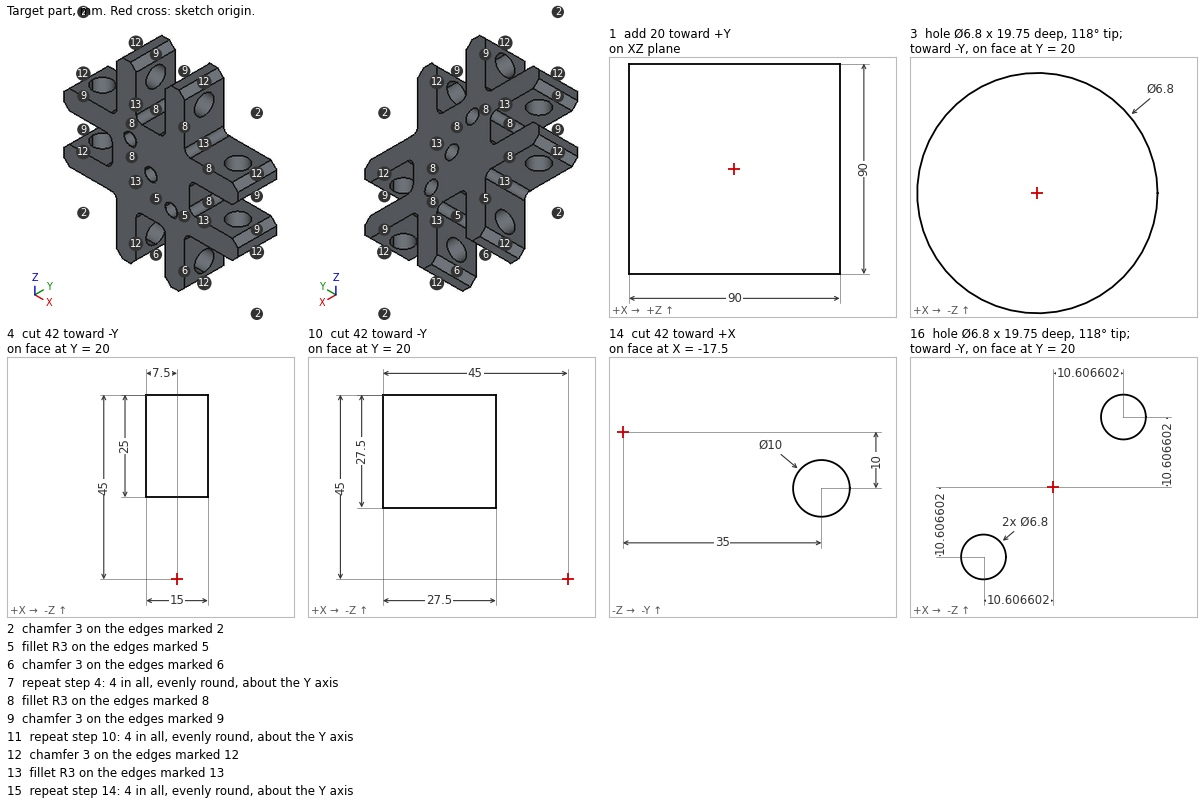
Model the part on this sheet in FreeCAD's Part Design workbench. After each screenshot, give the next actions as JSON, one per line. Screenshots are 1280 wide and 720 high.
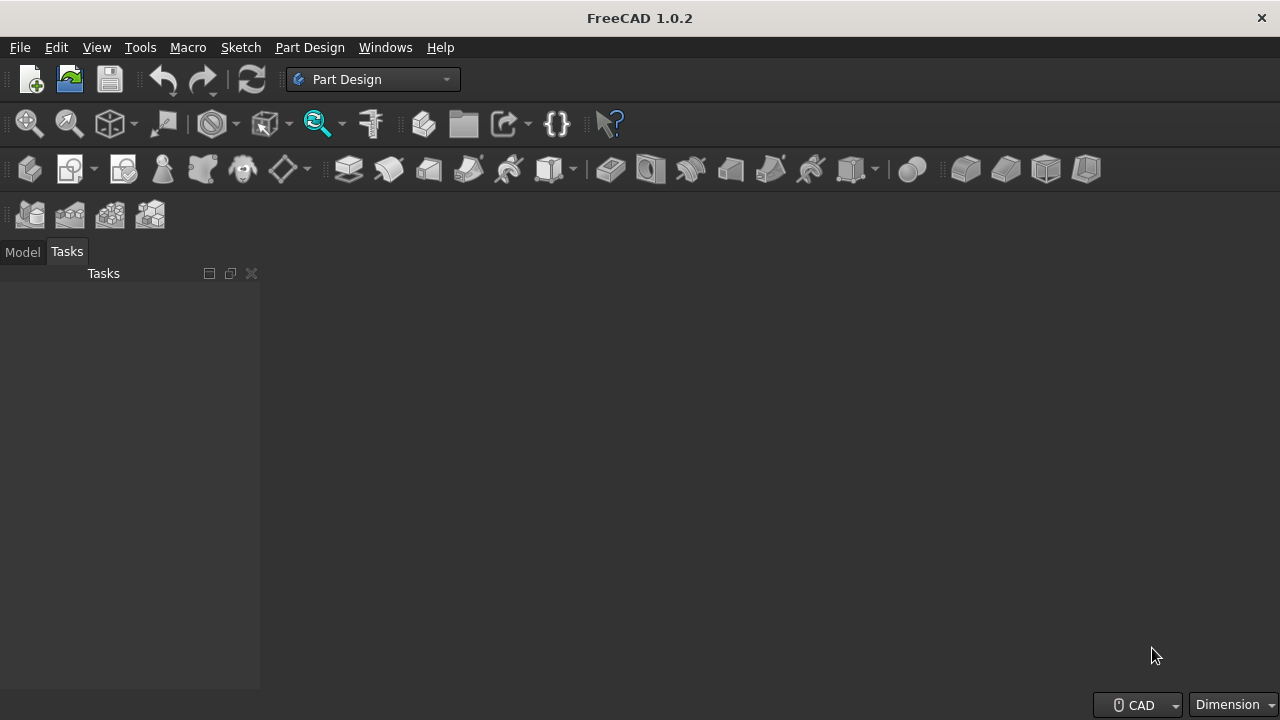
{"action": "left_click", "coordinate": [30, 80]}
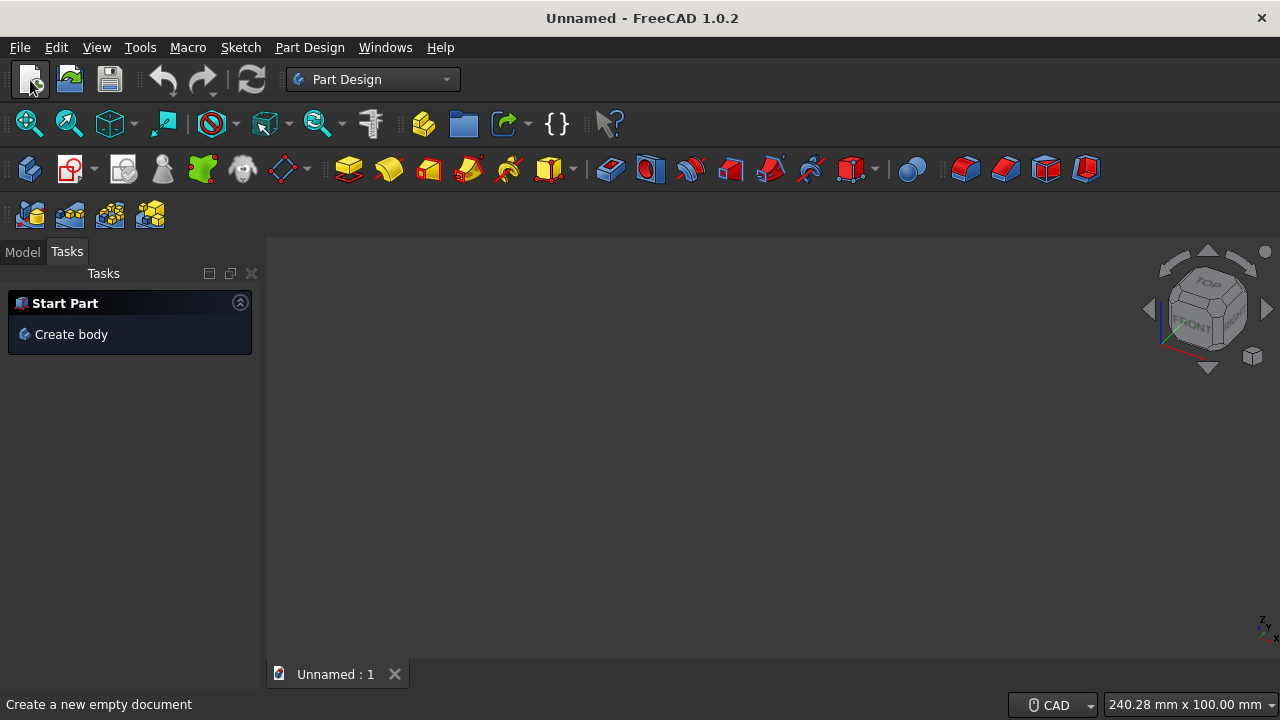
{"action": "left_click", "coordinate": [70, 170]}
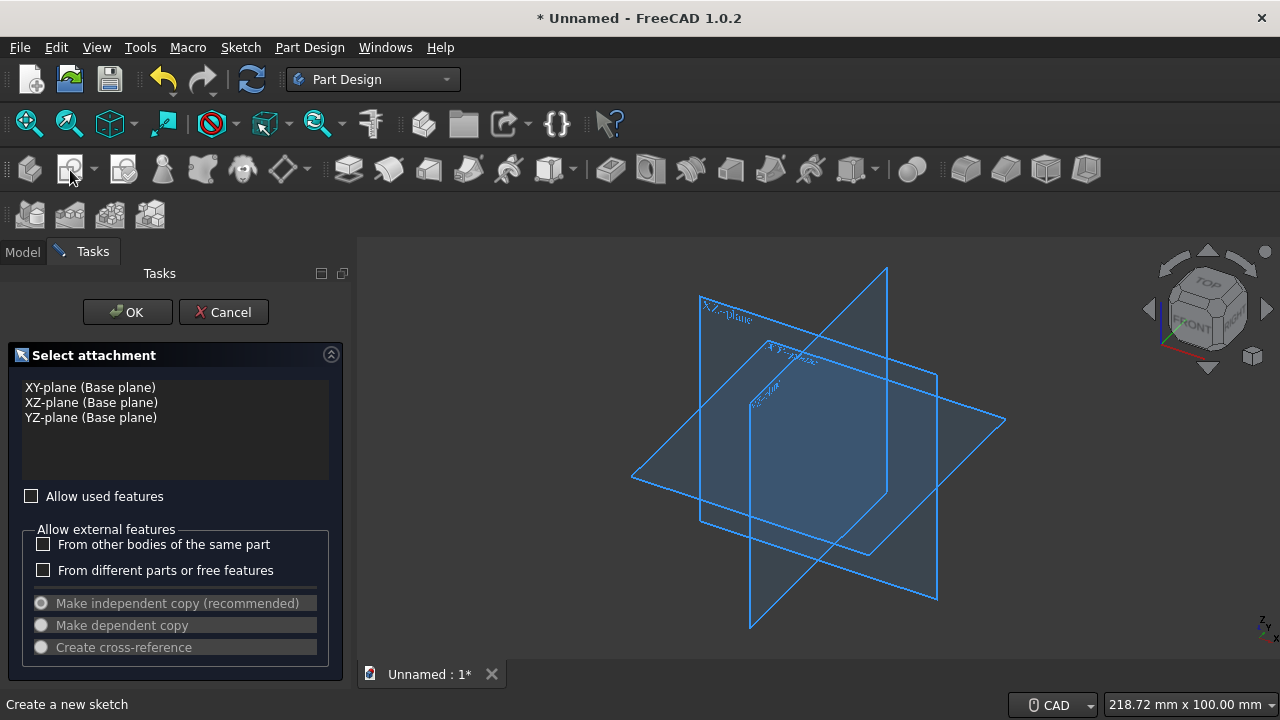
{"action": "left_click", "coordinate": [82, 402]}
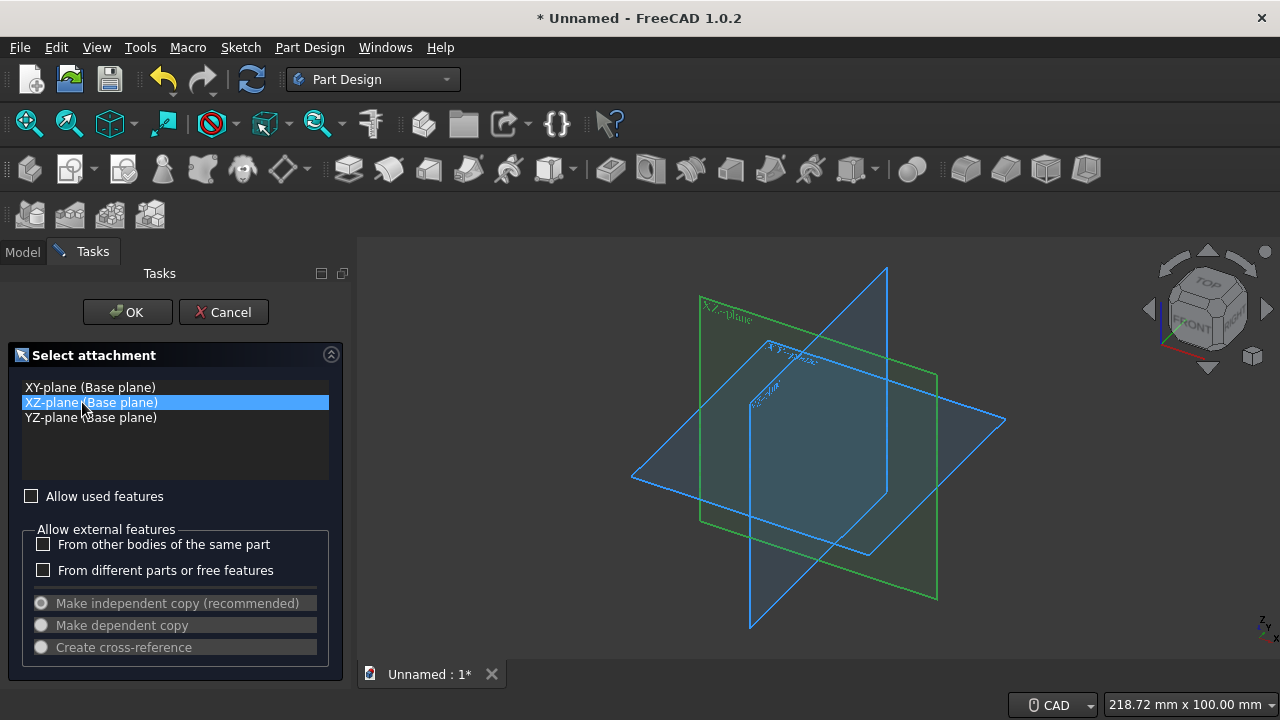
{"action": "left_click", "coordinate": [128, 312]}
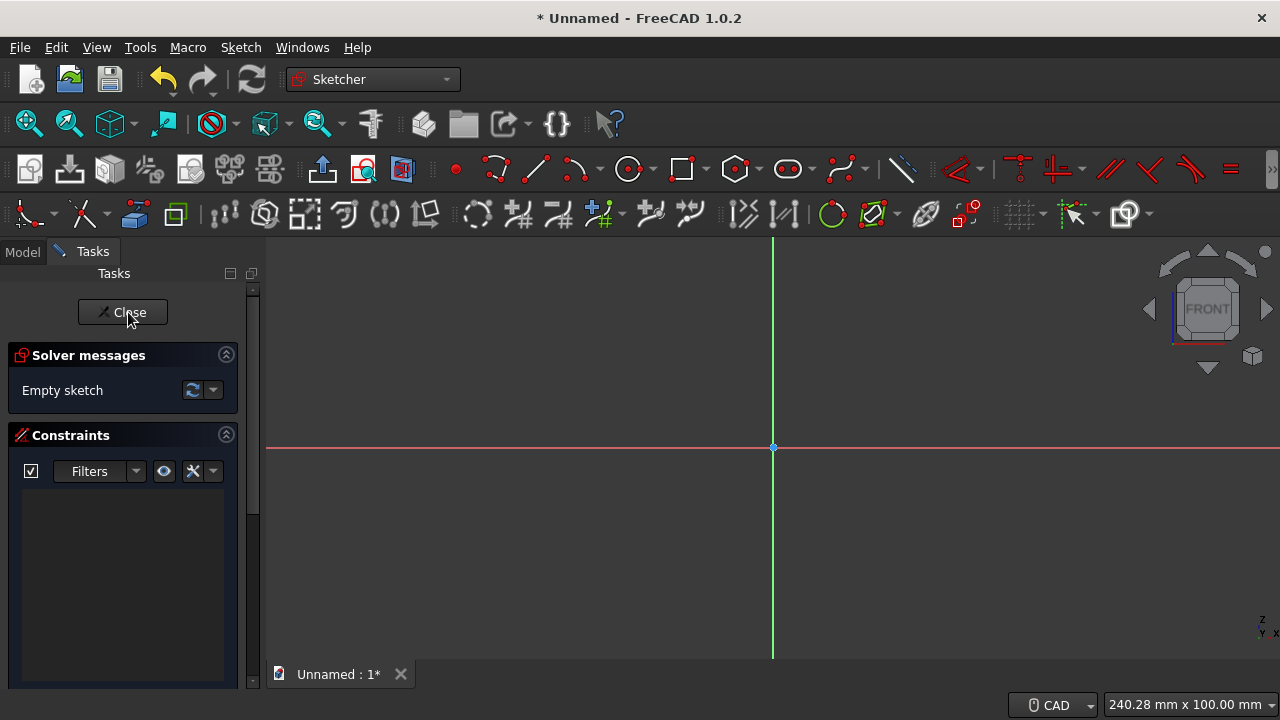
{"action": "scroll", "coordinate": [565, 448], "scroll_direction": "down", "scroll_amount": 2}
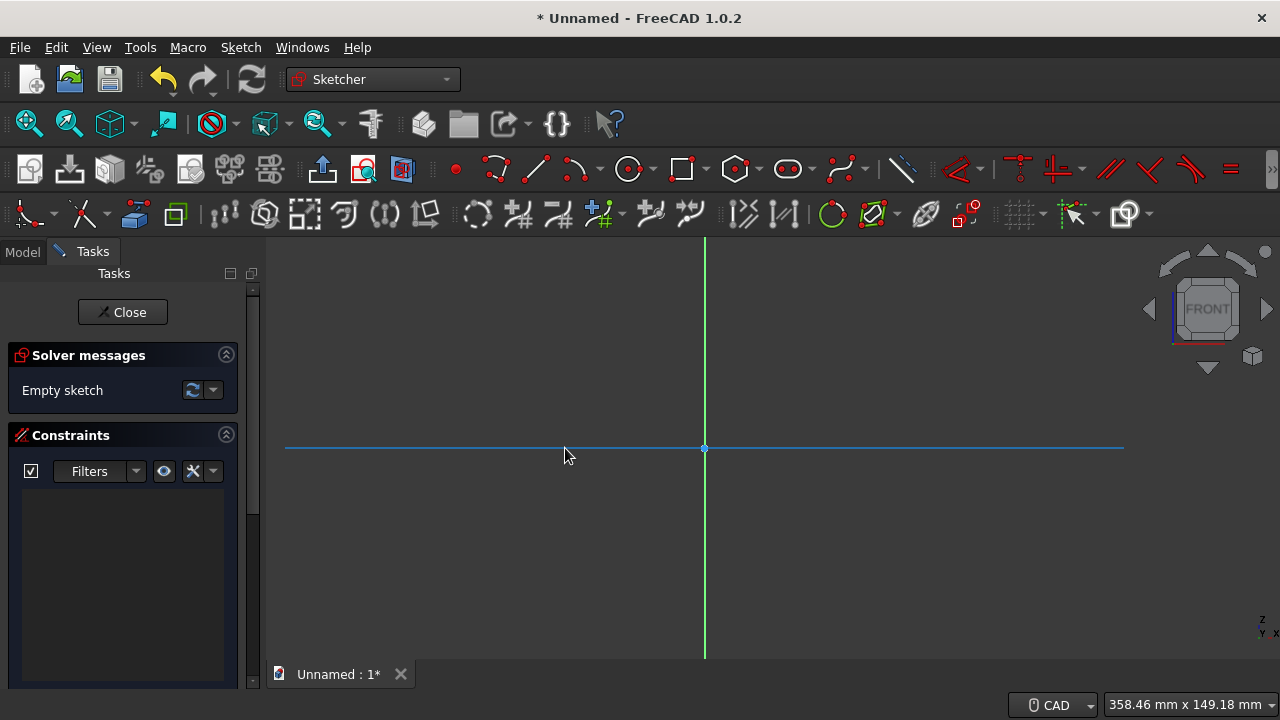
{"action": "left_click", "coordinate": [708, 170]}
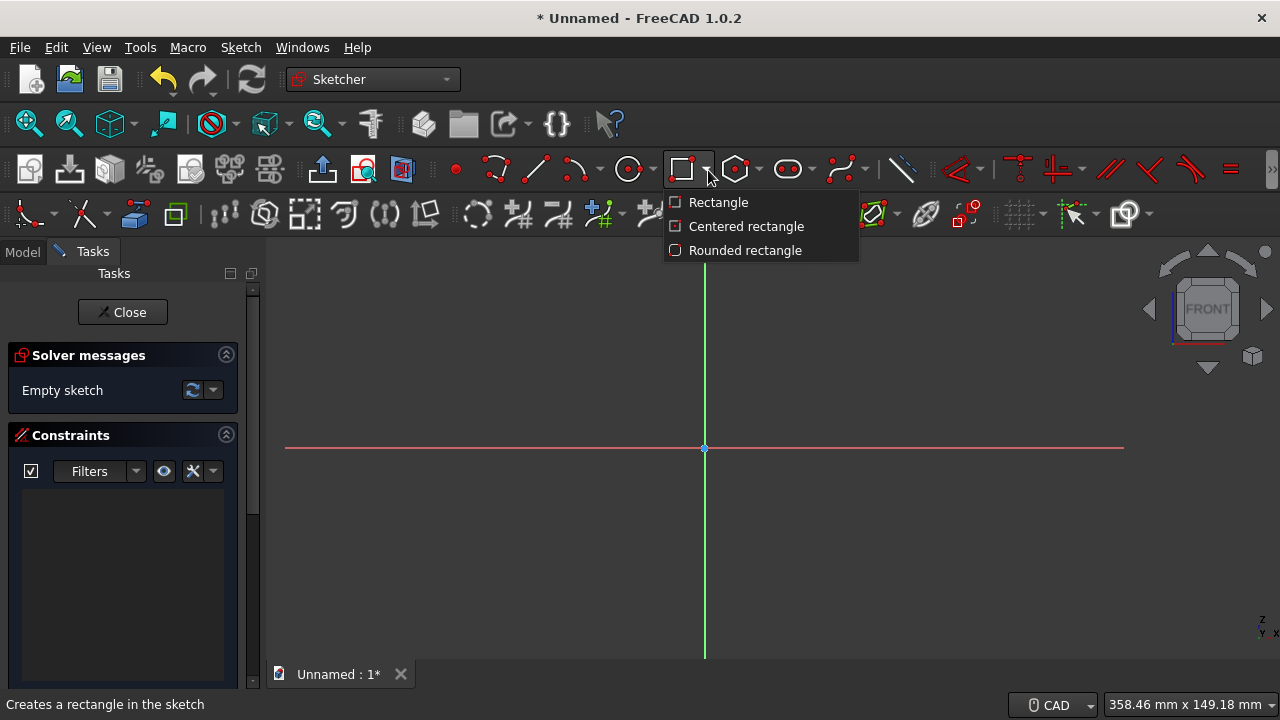
{"action": "left_click", "coordinate": [762, 226]}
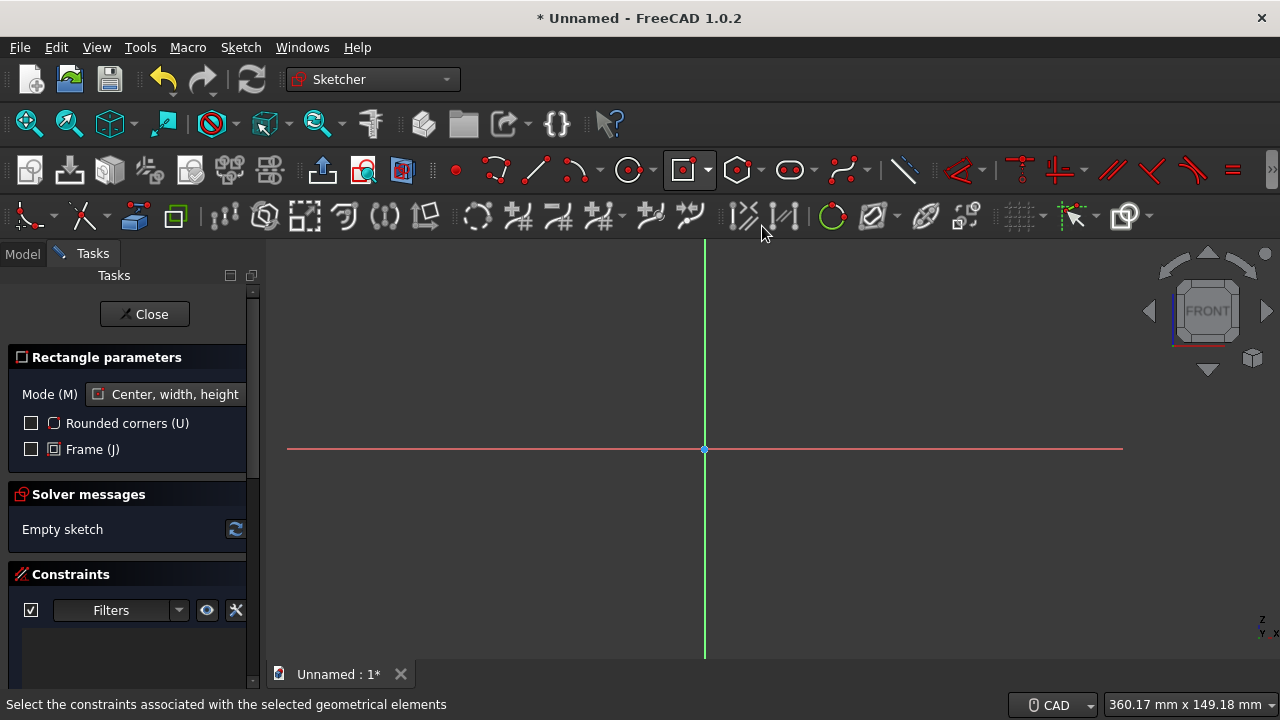
{"action": "left_click", "coordinate": [705, 449]}
{"action": "left_click", "coordinate": [832, 322]}
{"action": "key", "text": "Escape"}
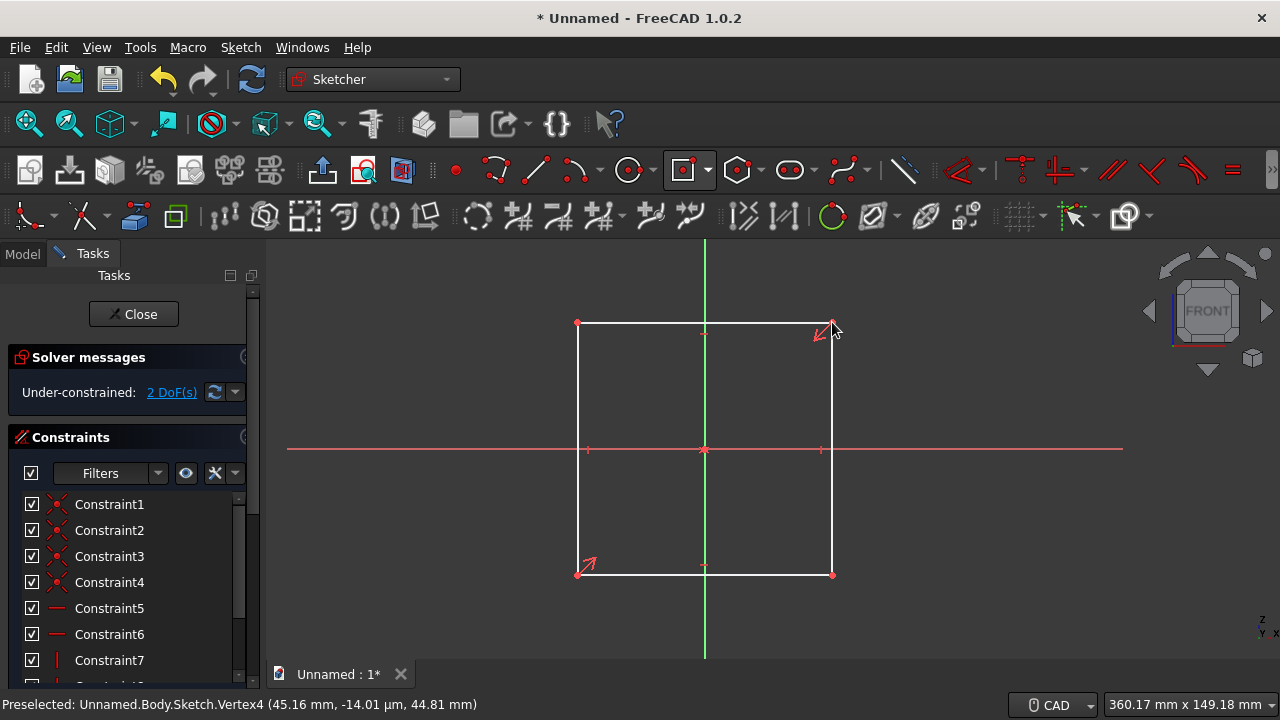
{"action": "left_click", "coordinate": [958, 170]}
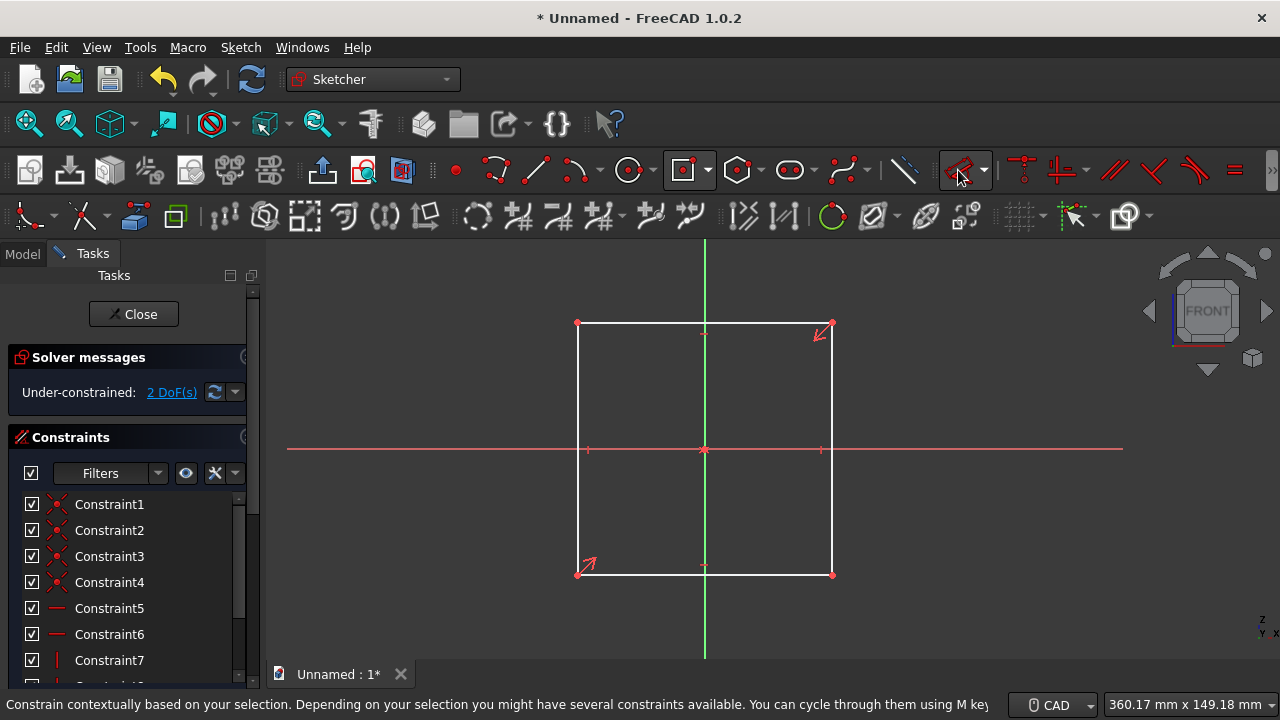
{"action": "left_click", "coordinate": [654, 575]}
{"action": "left_click", "coordinate": [646, 609]}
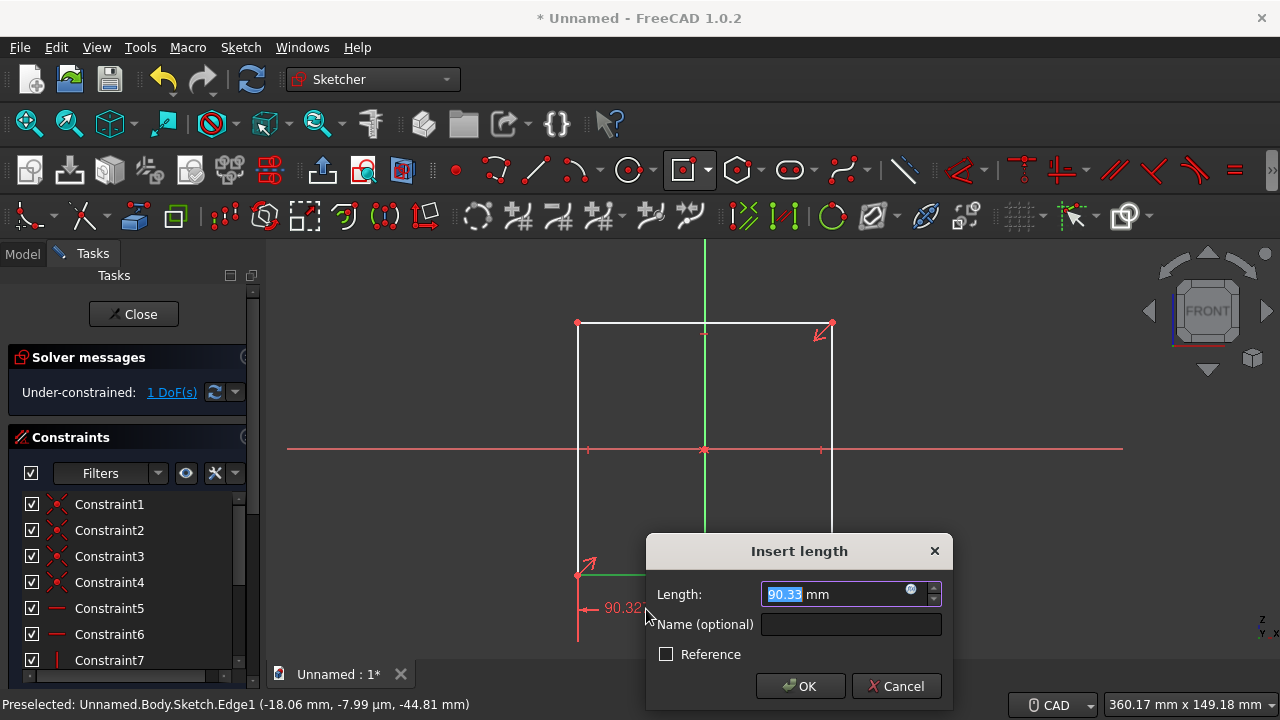
{"action": "type", "text": "90"}
{"action": "key", "text": "Return"}